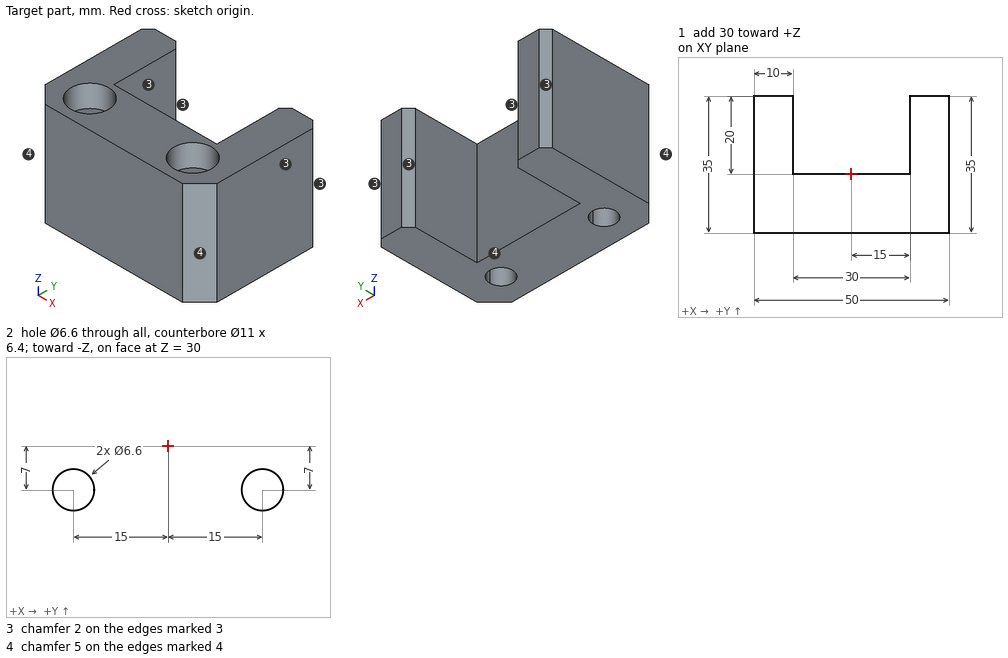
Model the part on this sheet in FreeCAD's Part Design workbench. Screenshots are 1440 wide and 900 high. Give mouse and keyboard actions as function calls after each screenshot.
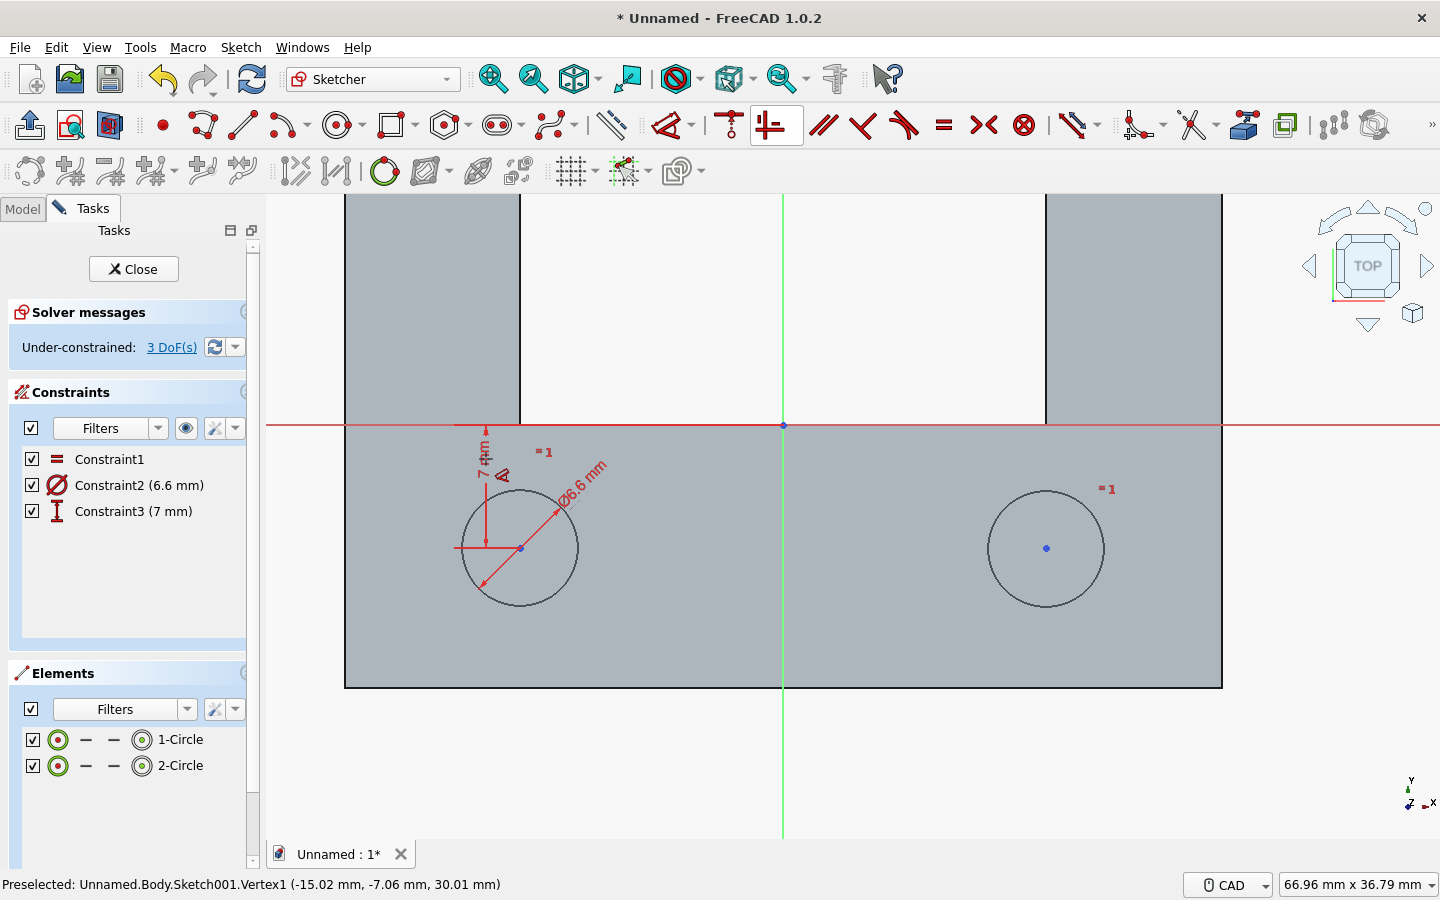
click(1046, 549)
click(1080, 459)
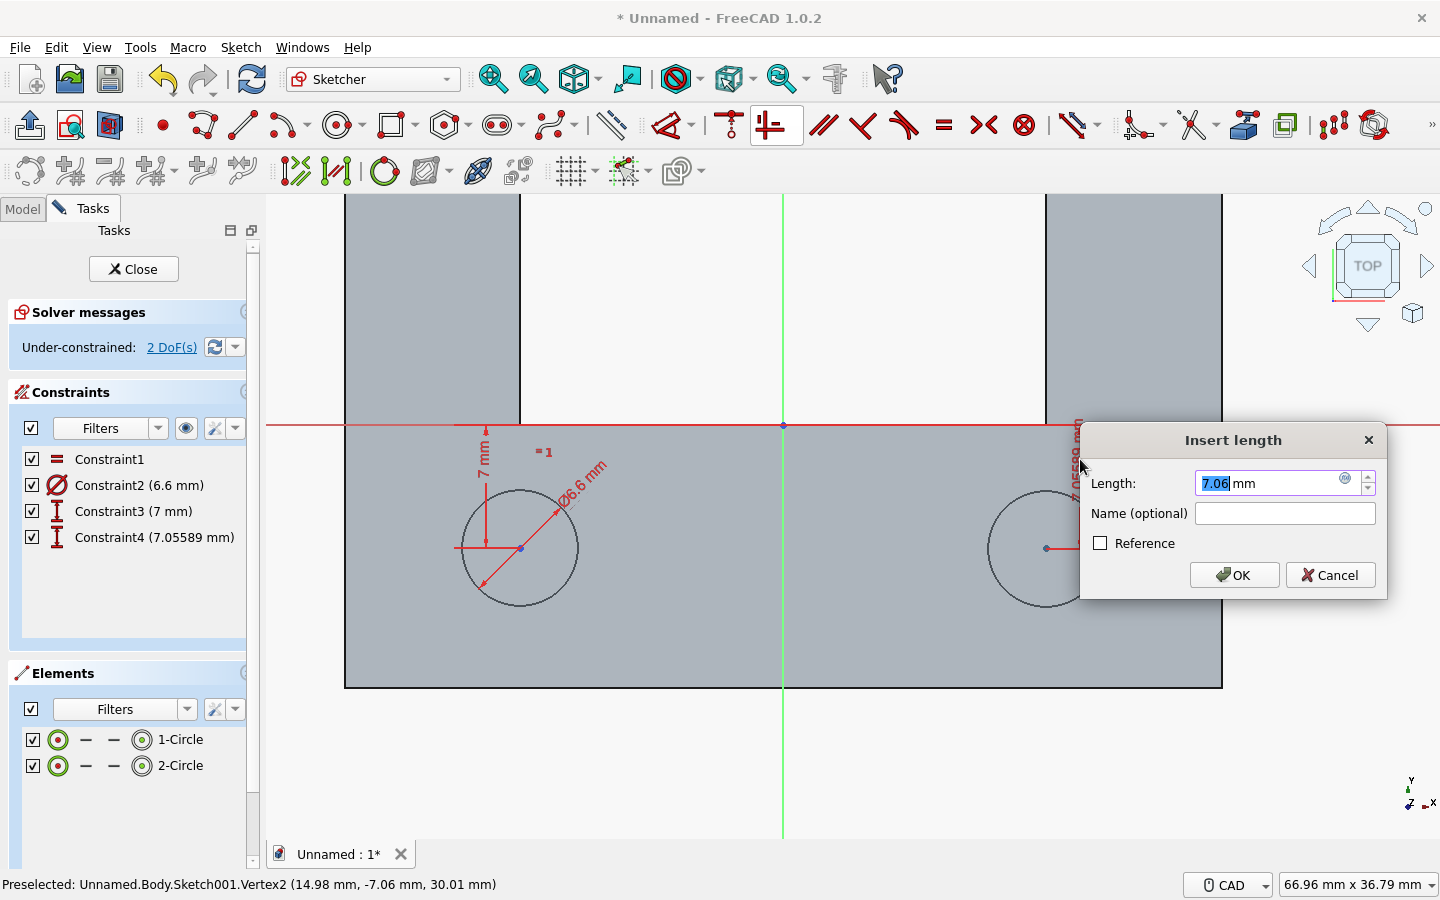
text(7)
key(Return)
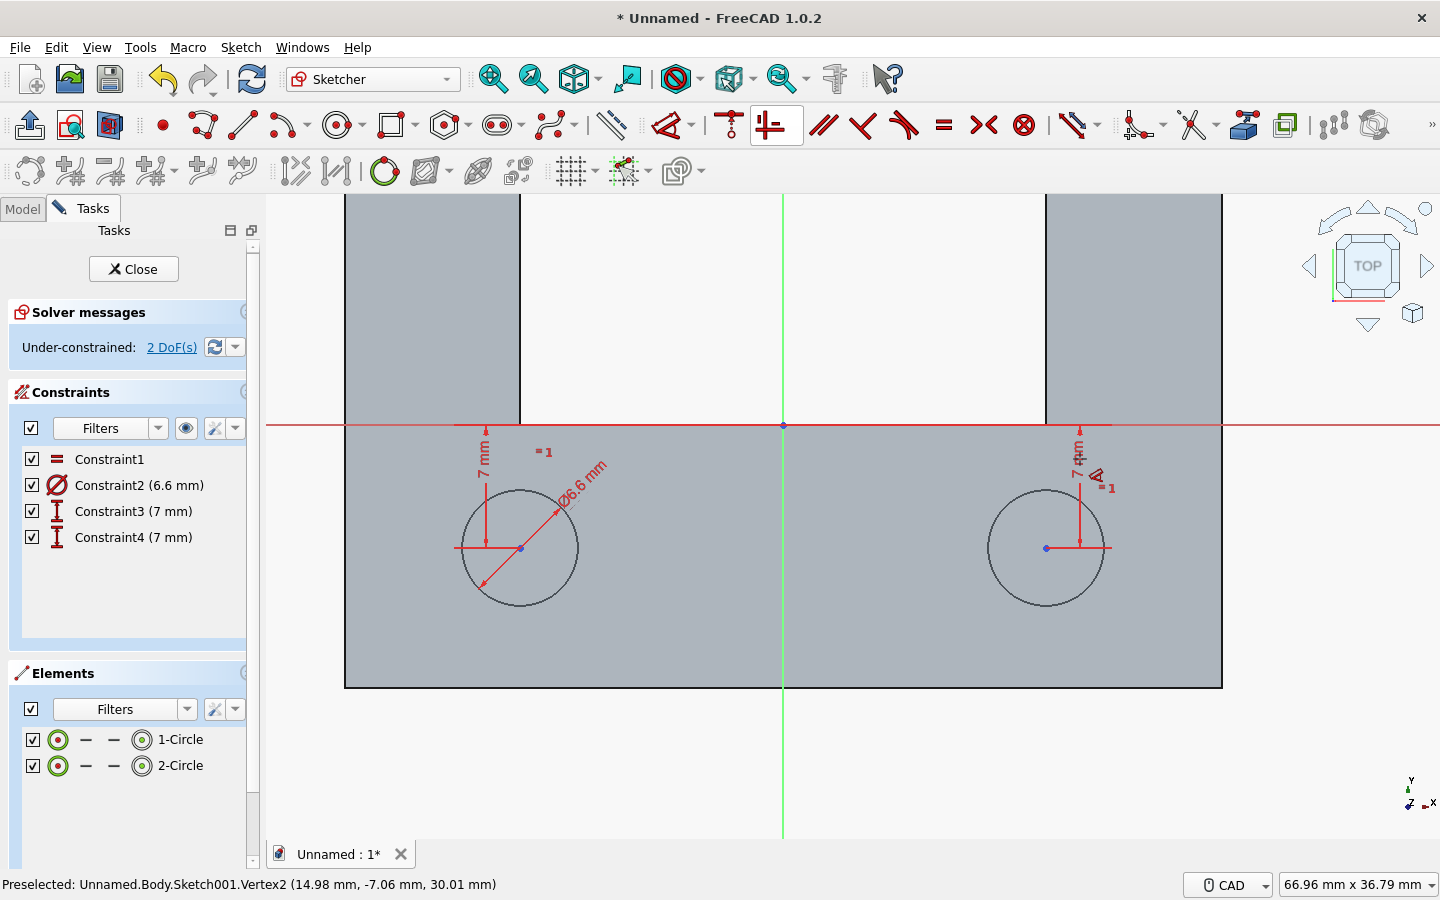
click(520, 548)
click(652, 391)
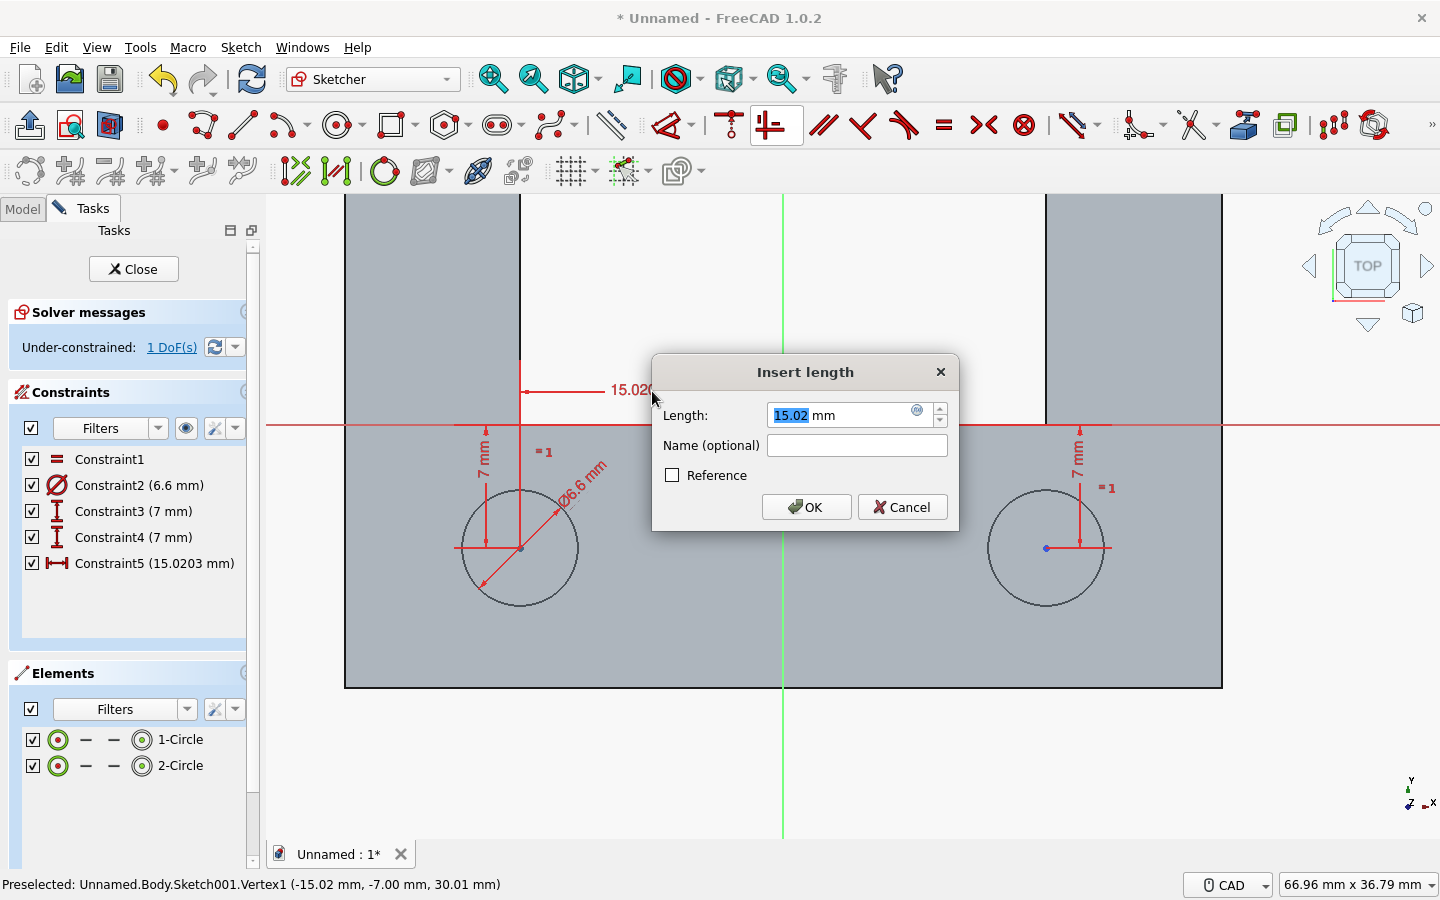
text(15)
key(Return)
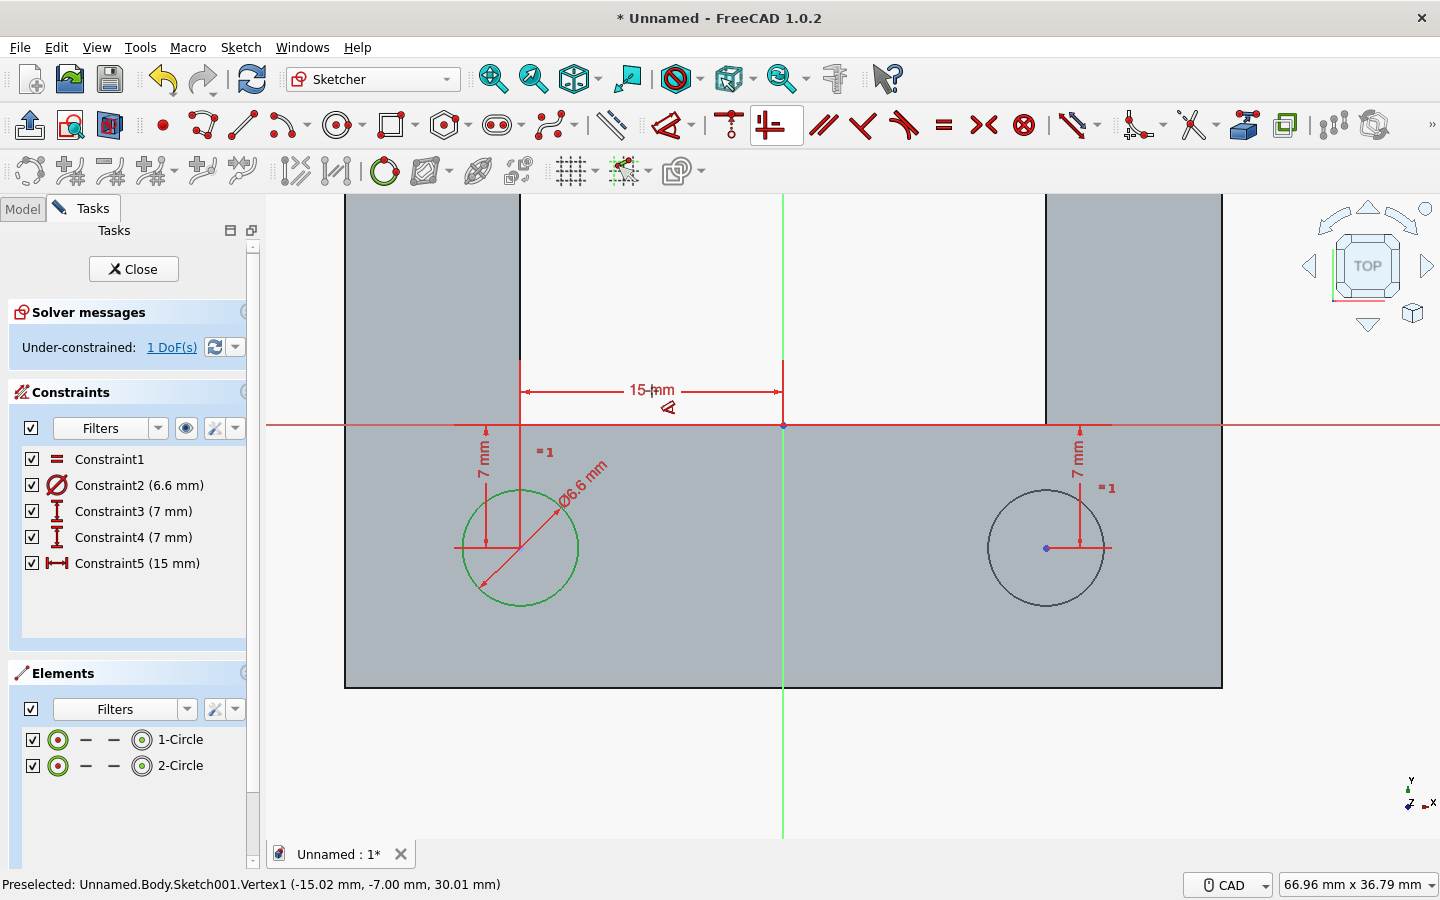
click(1046, 548)
click(915, 391)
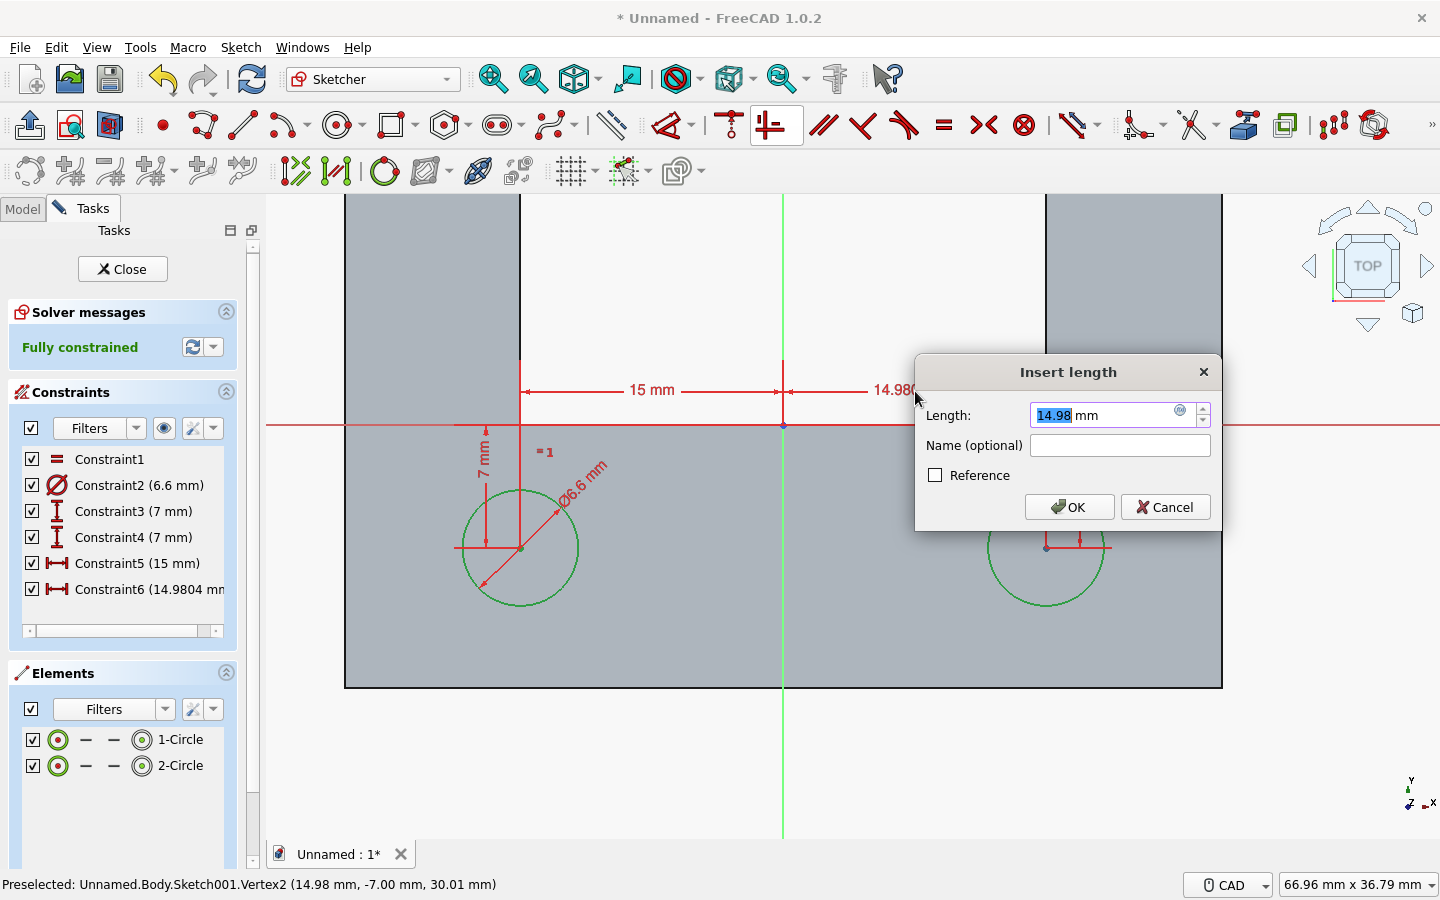
text(15)
key(Return)
key(Escape)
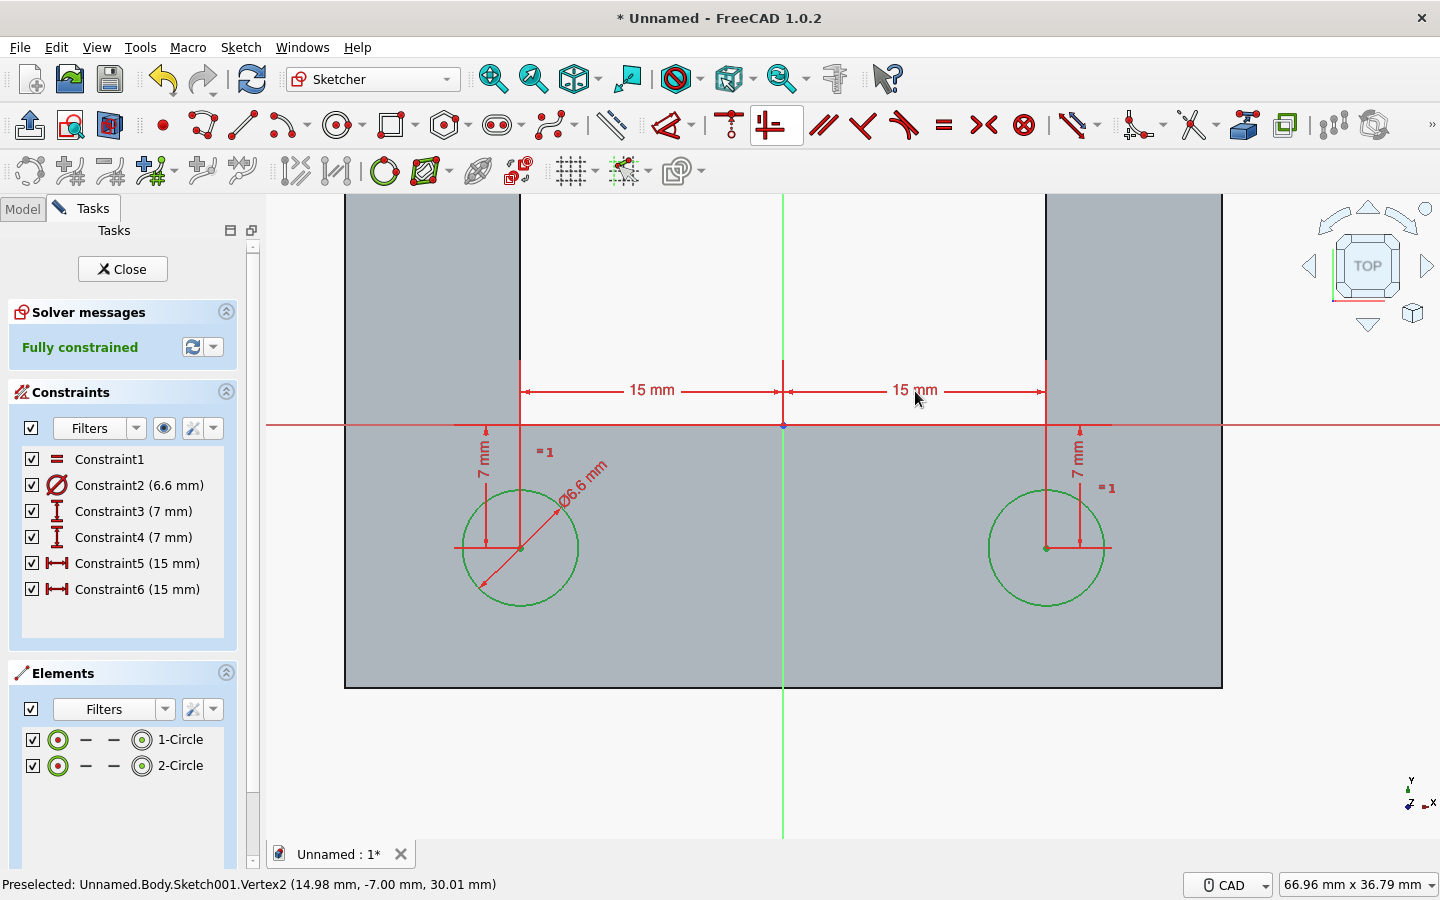
click(123, 269)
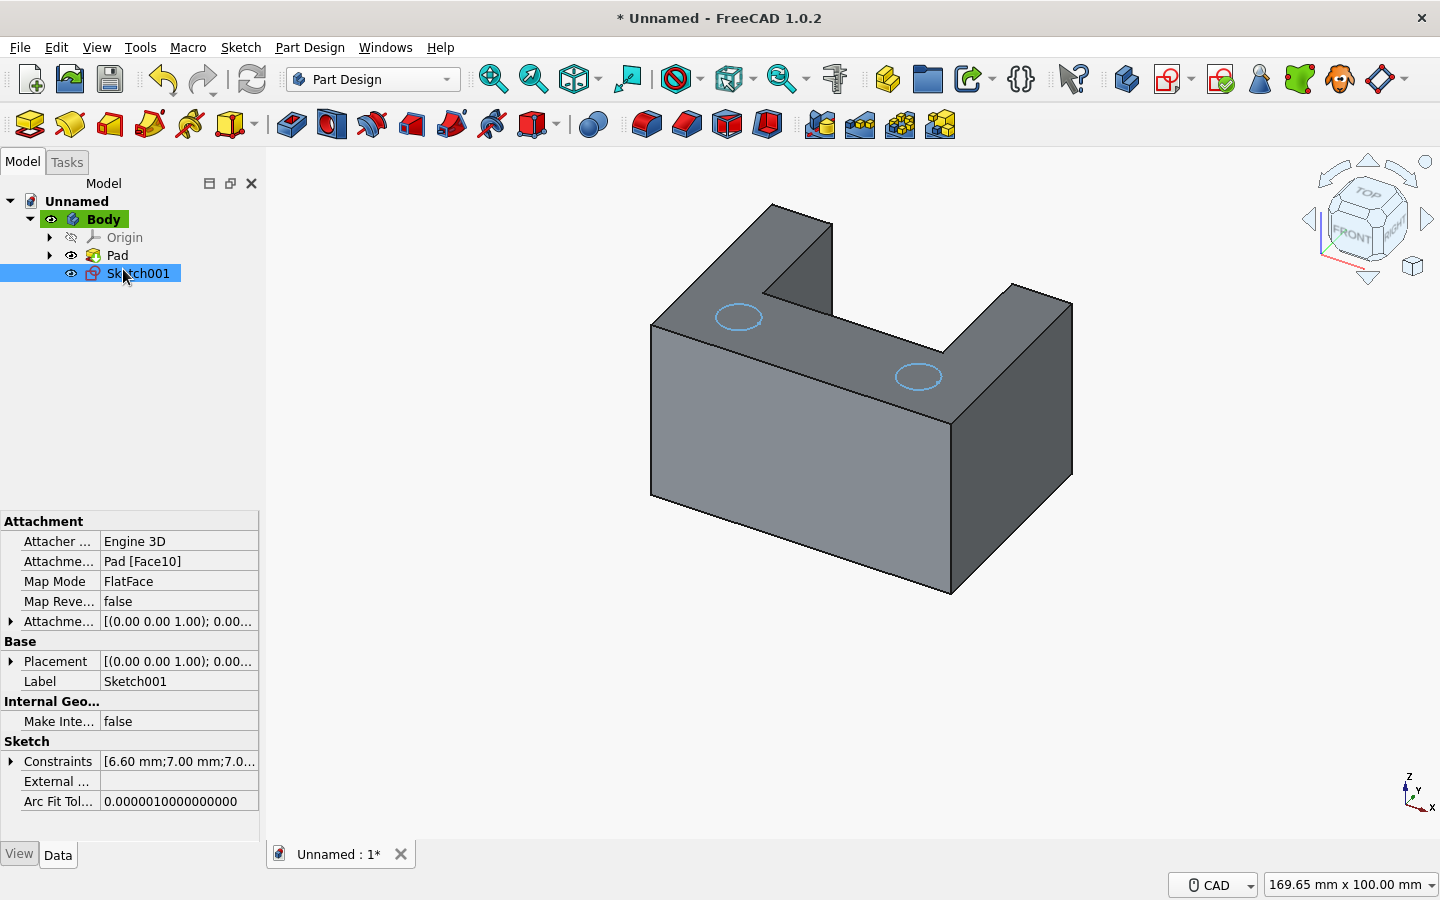
click(332, 124)